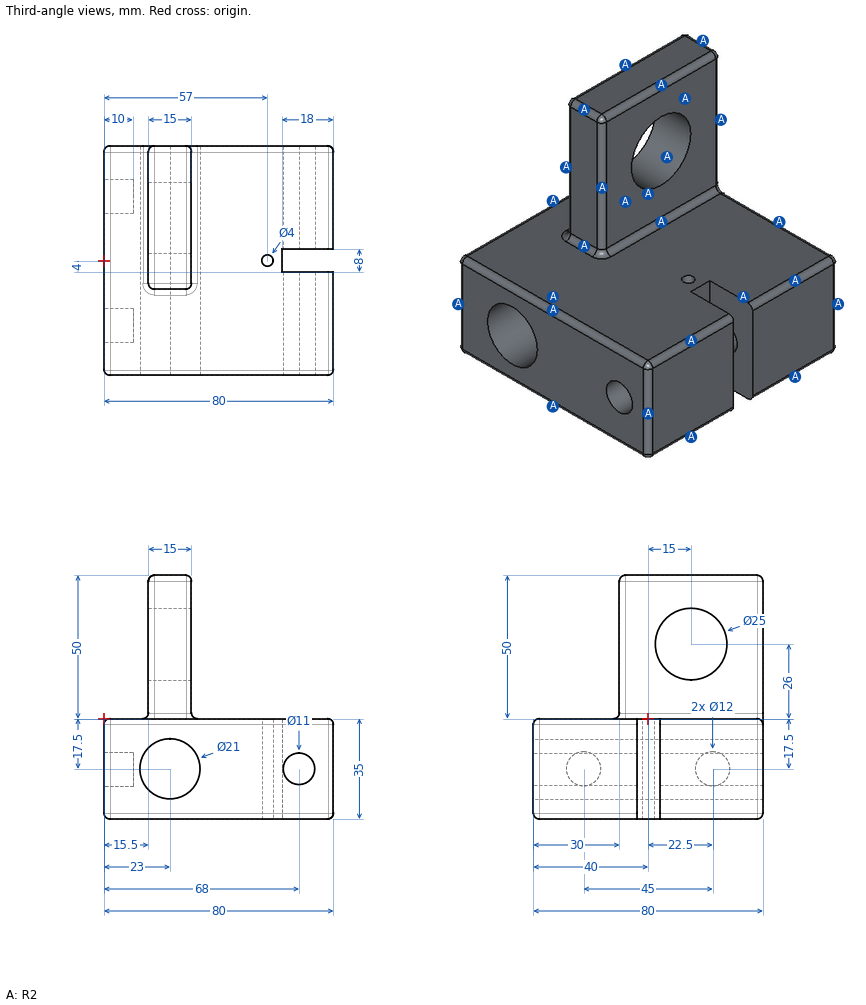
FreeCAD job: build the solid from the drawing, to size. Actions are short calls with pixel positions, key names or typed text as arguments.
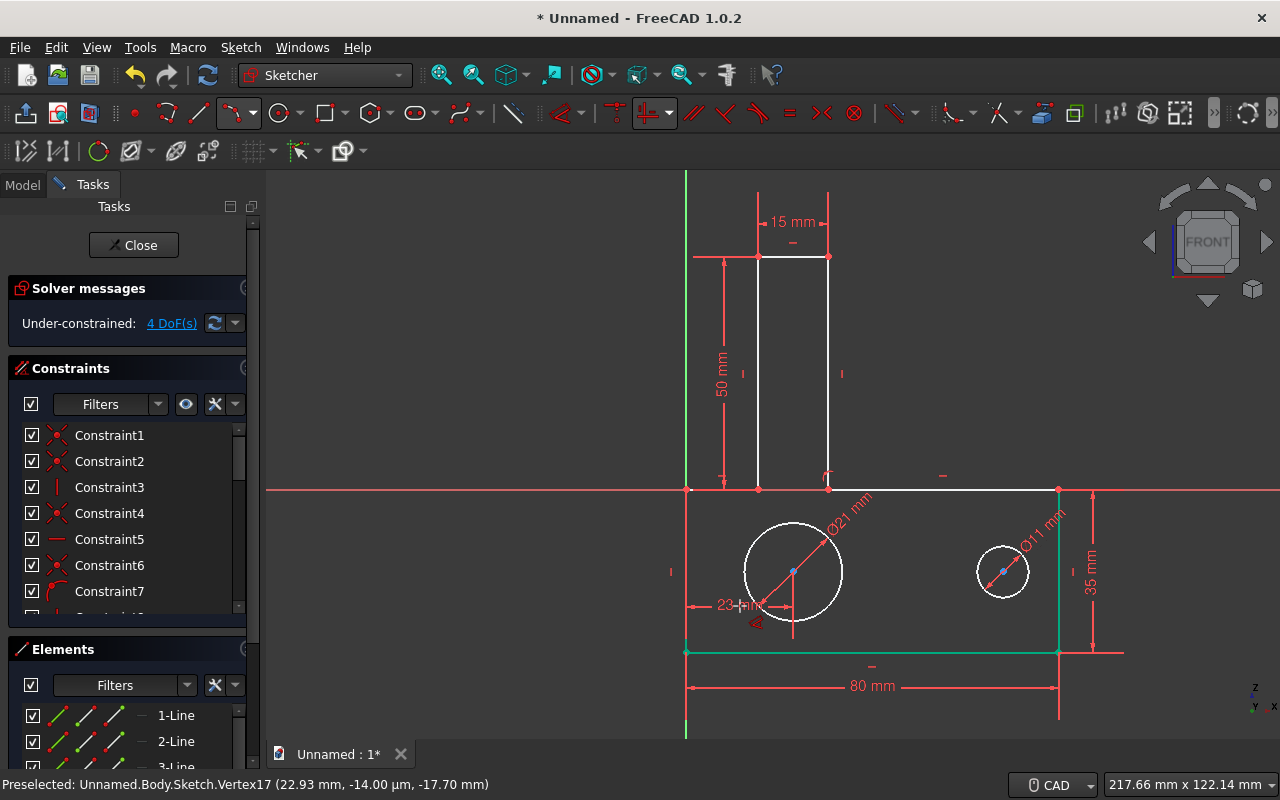
click(1003, 572)
click(917, 606)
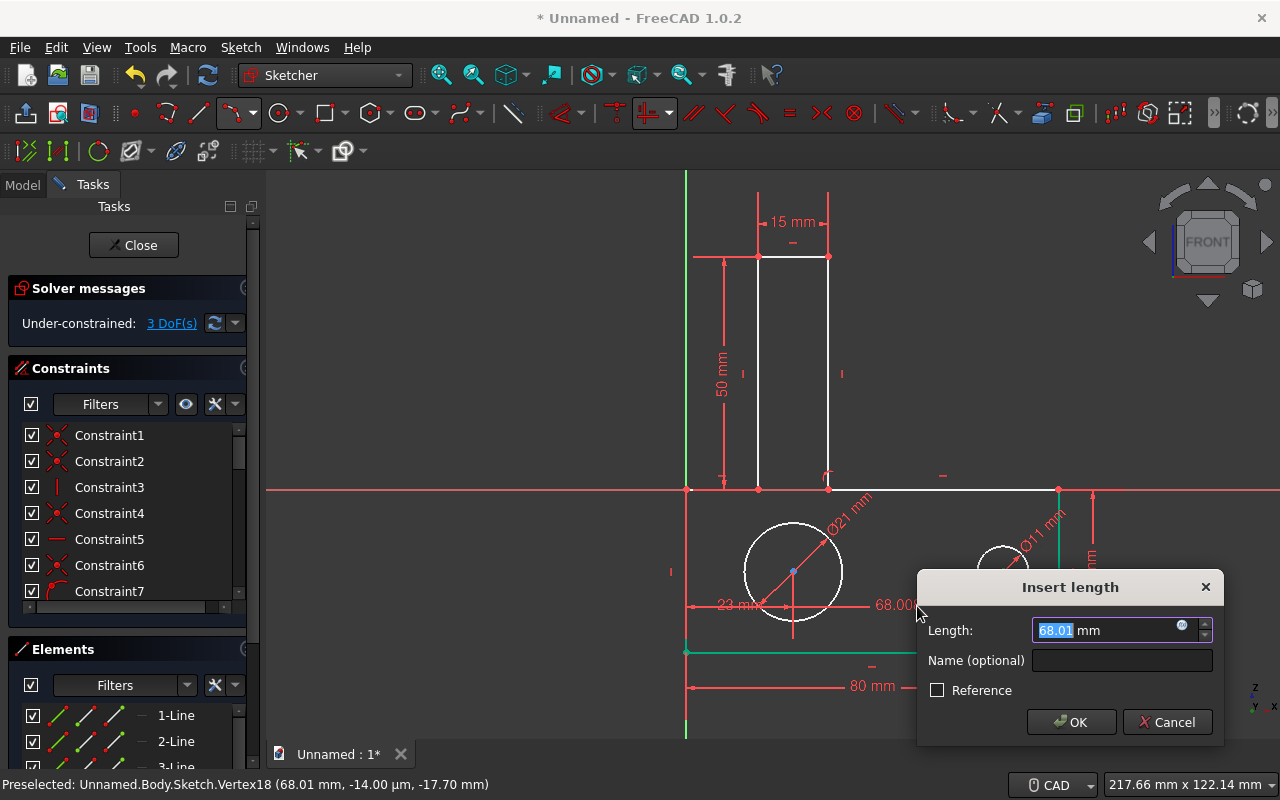
text(68)
key(Return)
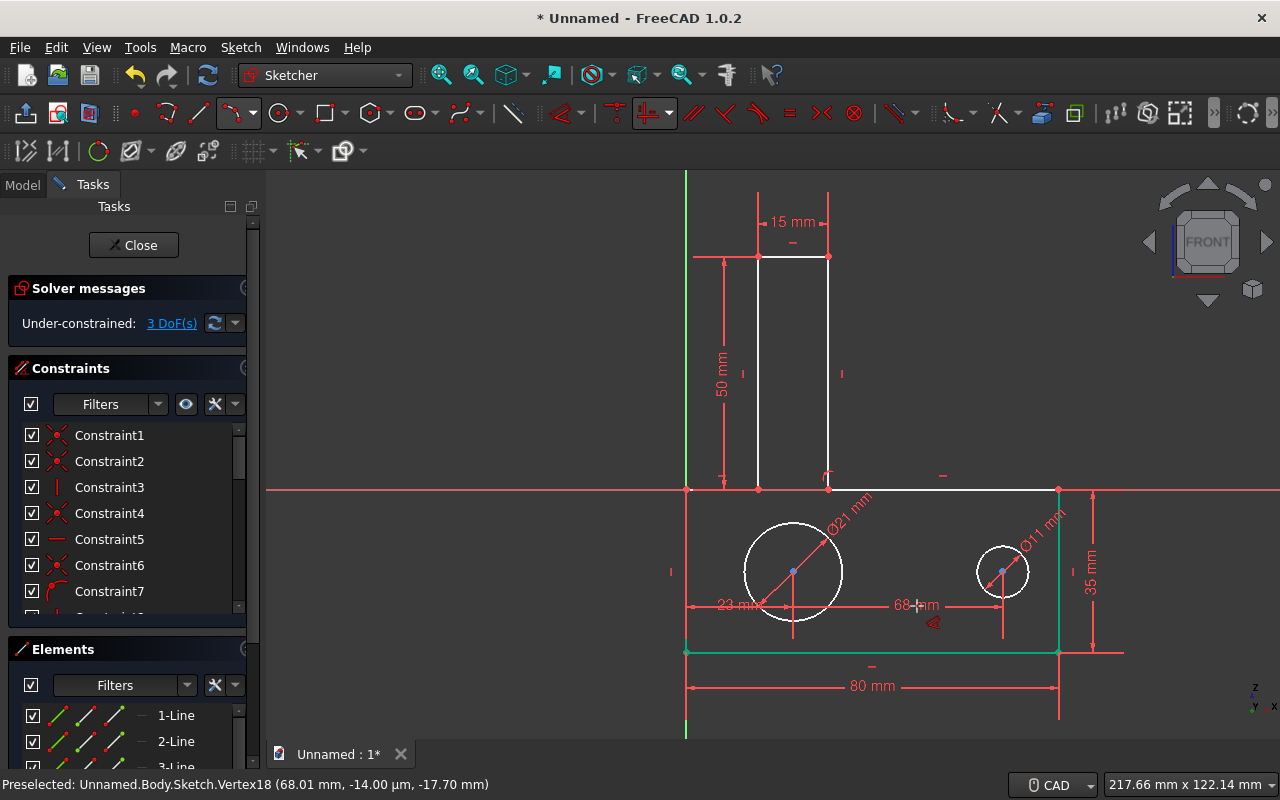
click(708, 490)
click(722, 524)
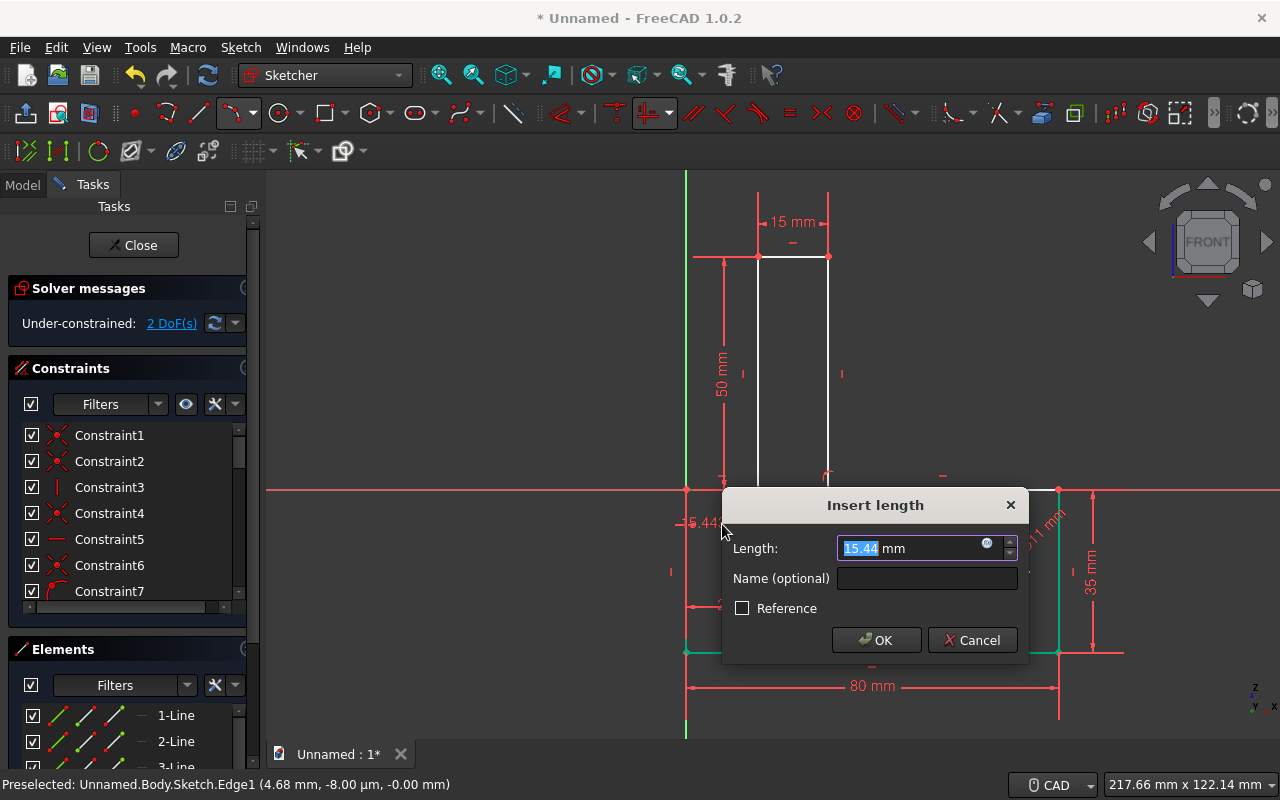
text(15.5)
key(Return)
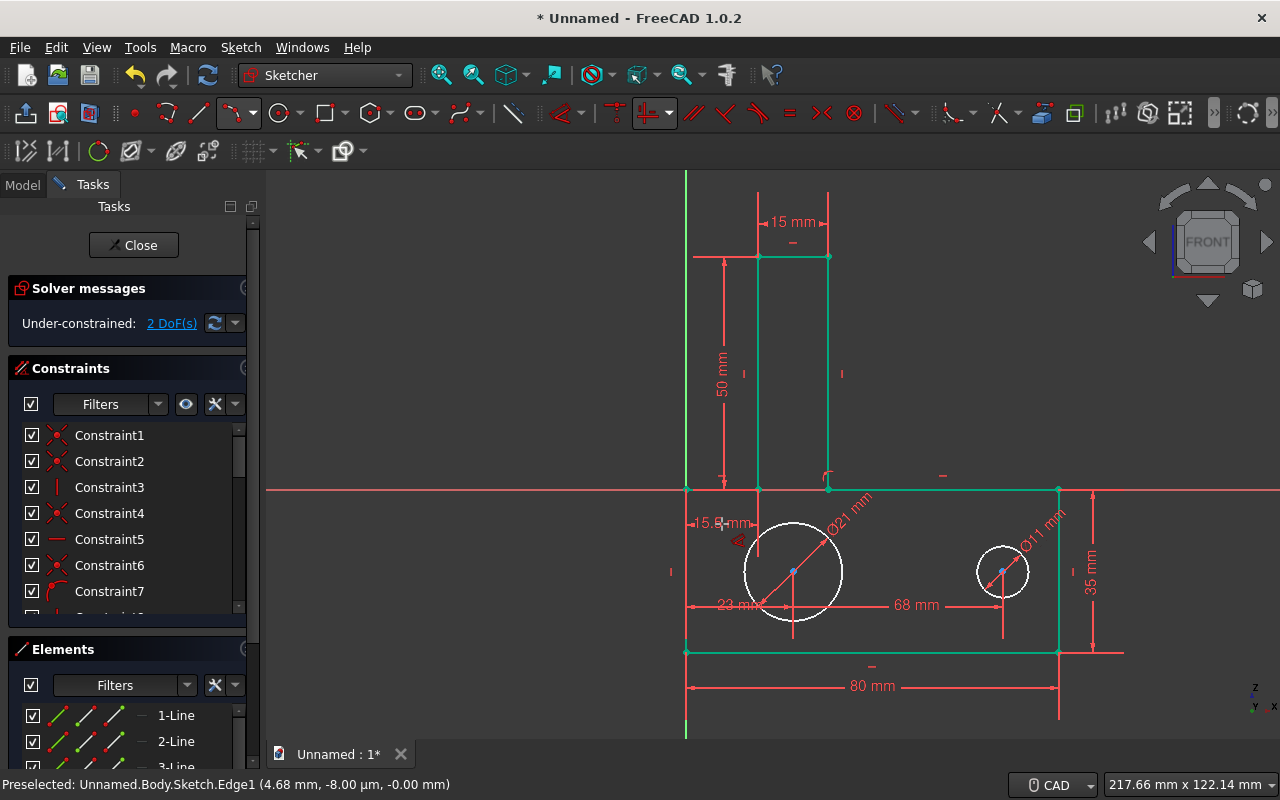
click(793, 572)
click(652, 550)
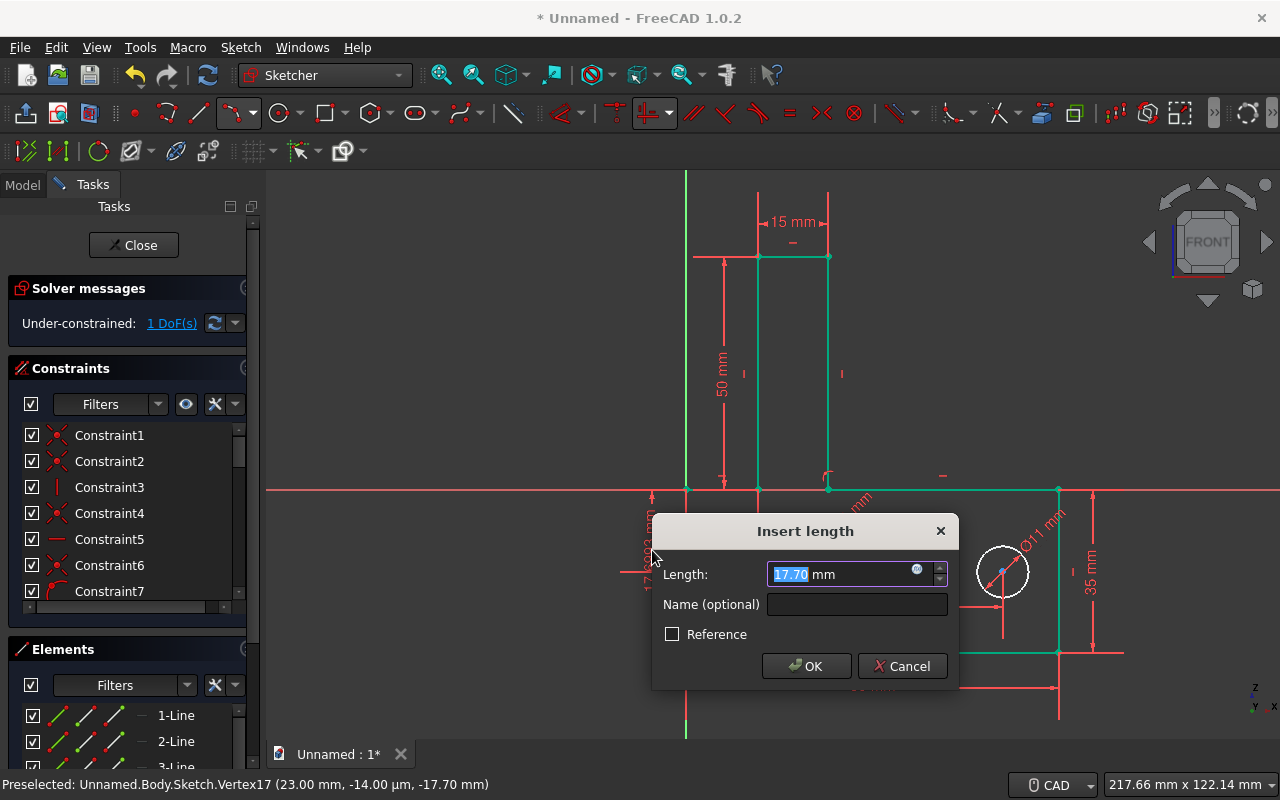
text(17.5)
key(Return)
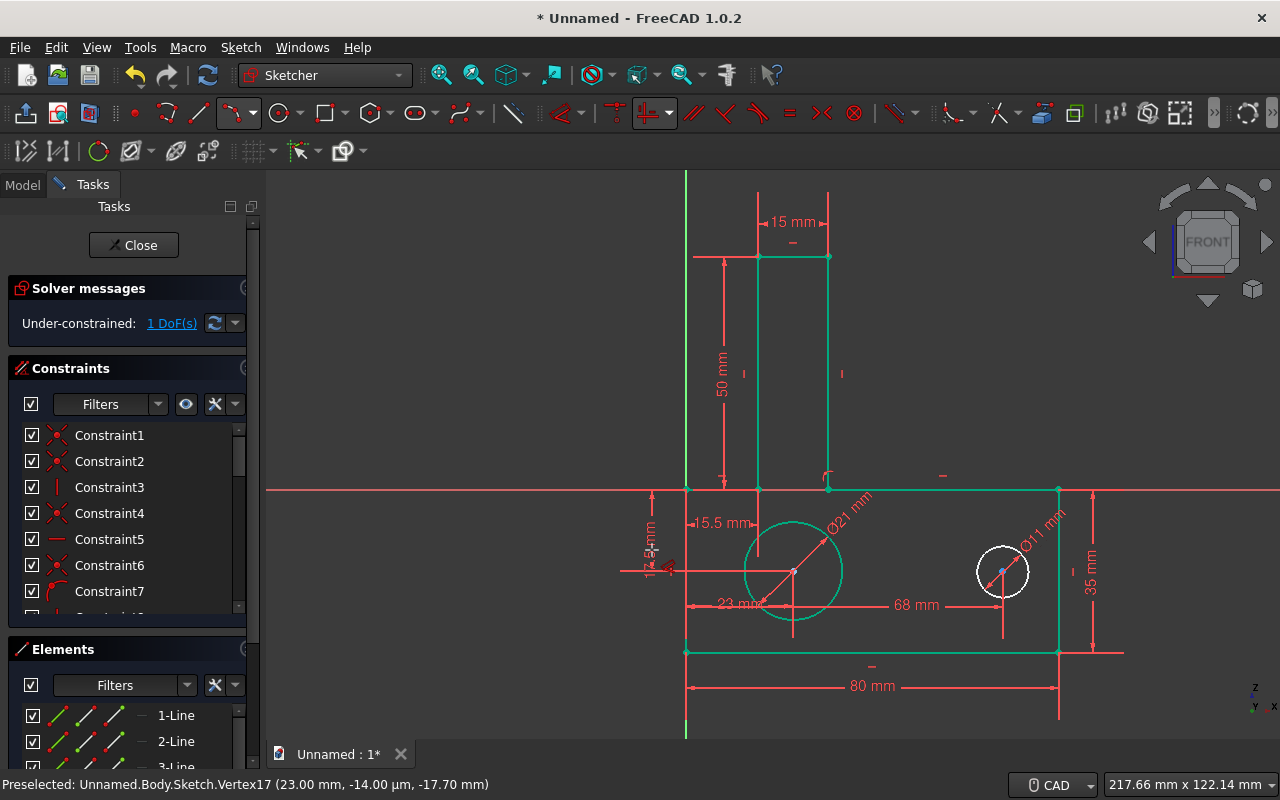
click(1003, 572)
click(628, 512)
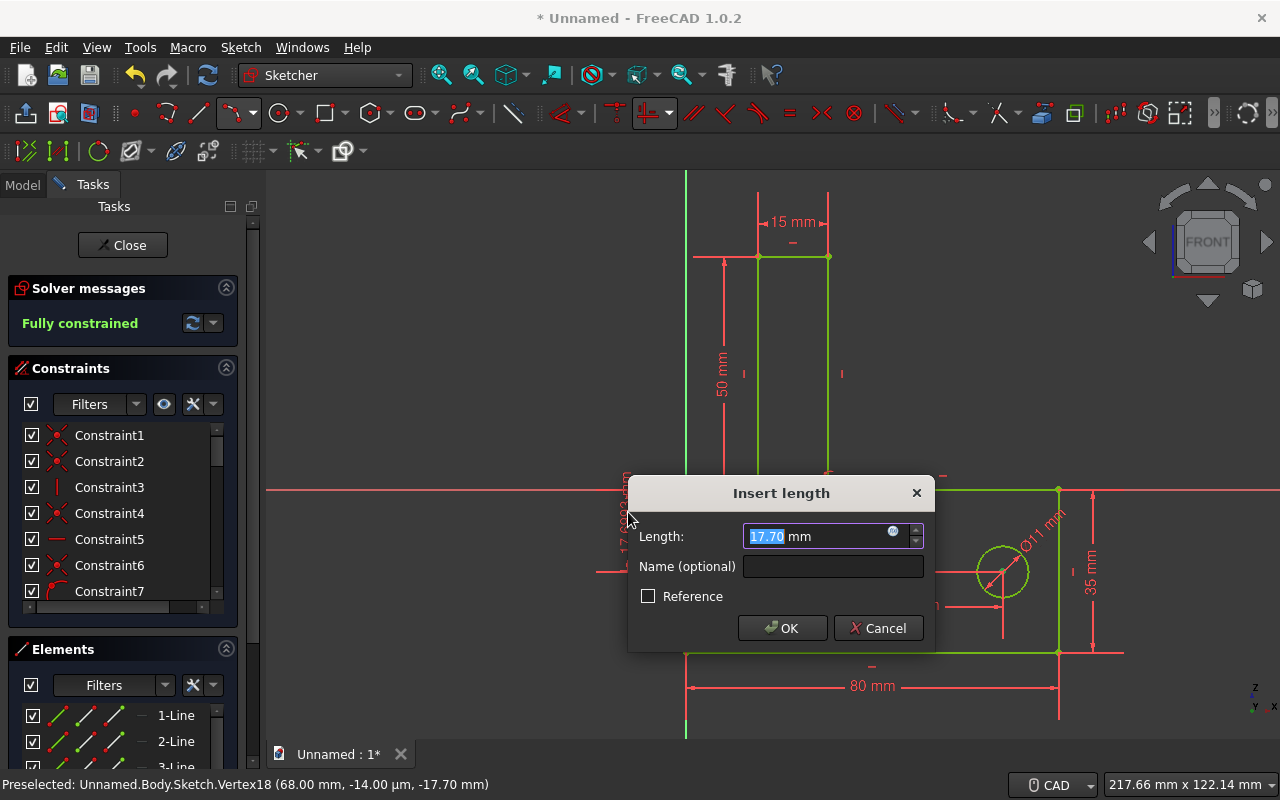
text(17.5)
key(Return)
key(Escape)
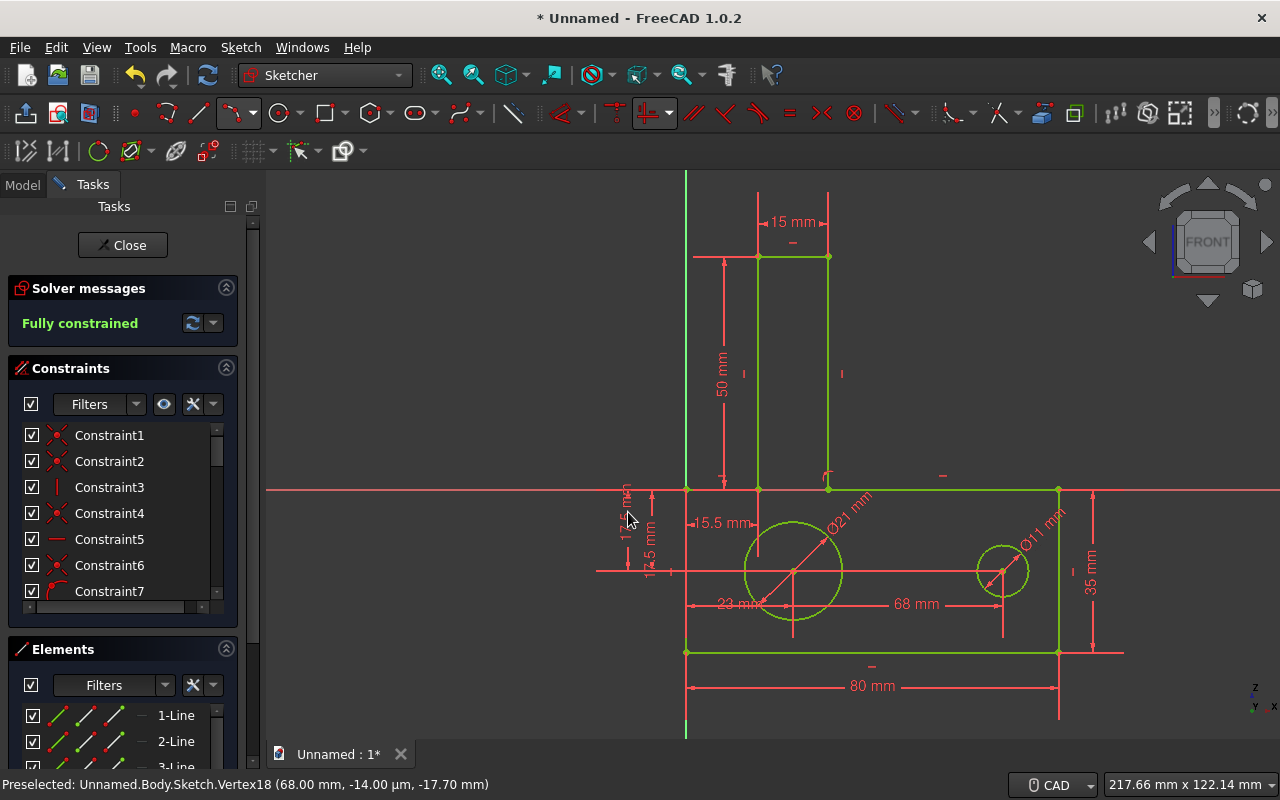
click(123, 245)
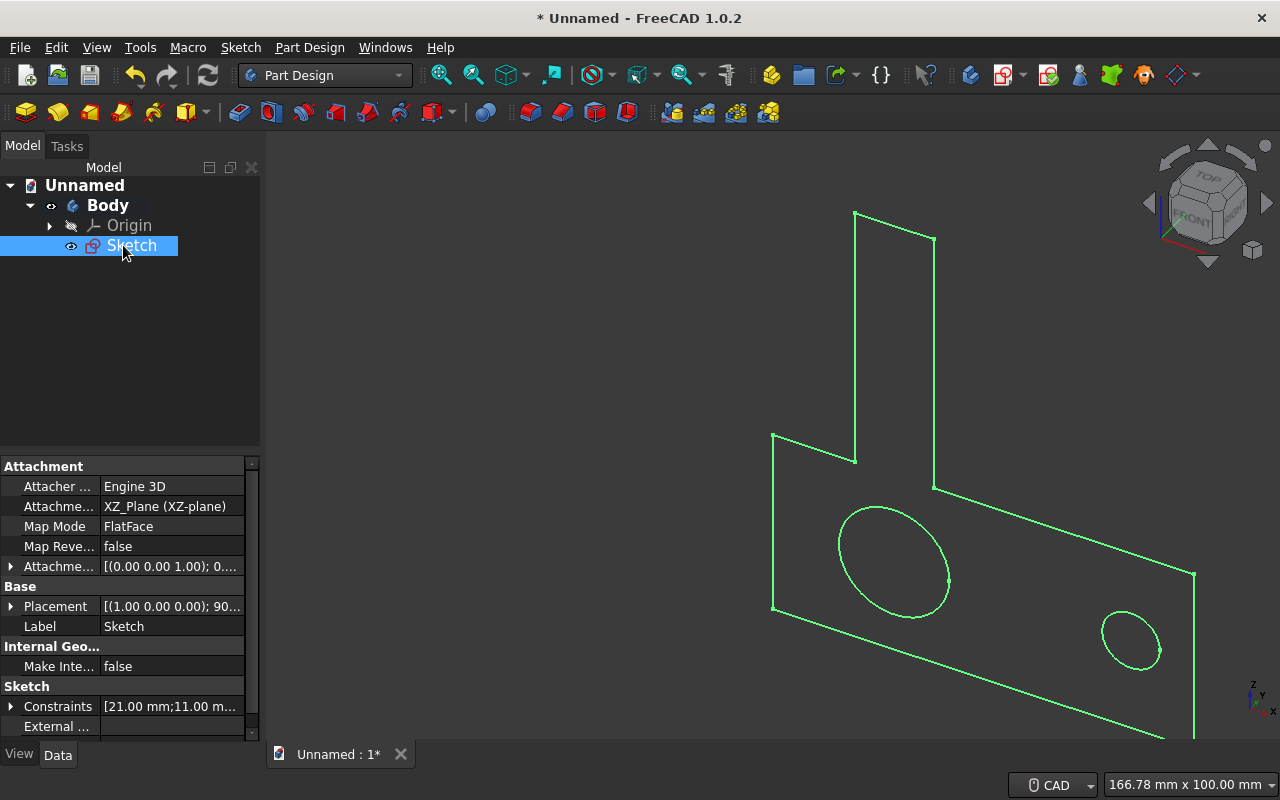
click(26, 112)